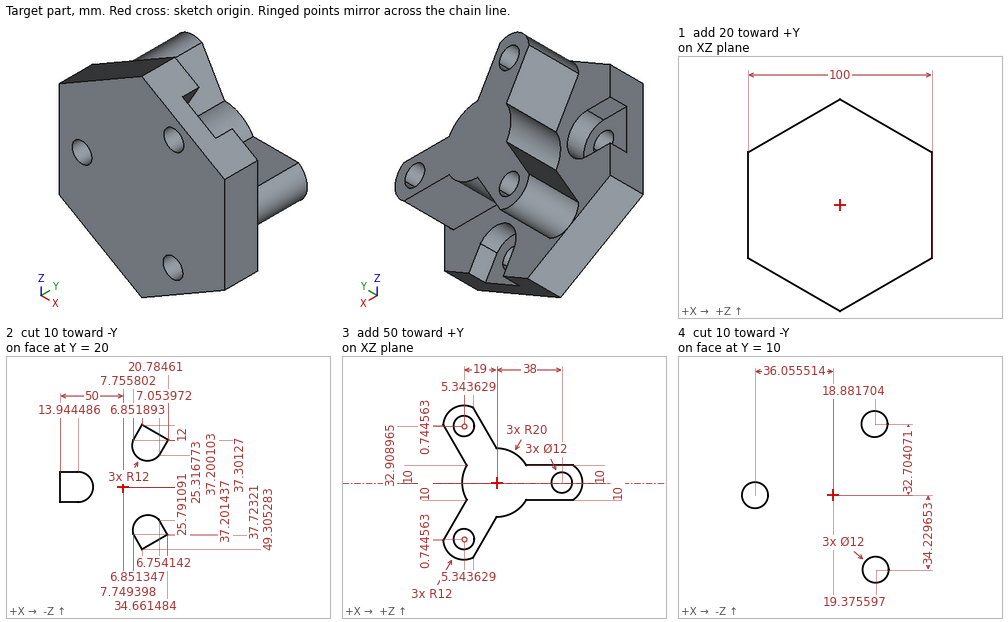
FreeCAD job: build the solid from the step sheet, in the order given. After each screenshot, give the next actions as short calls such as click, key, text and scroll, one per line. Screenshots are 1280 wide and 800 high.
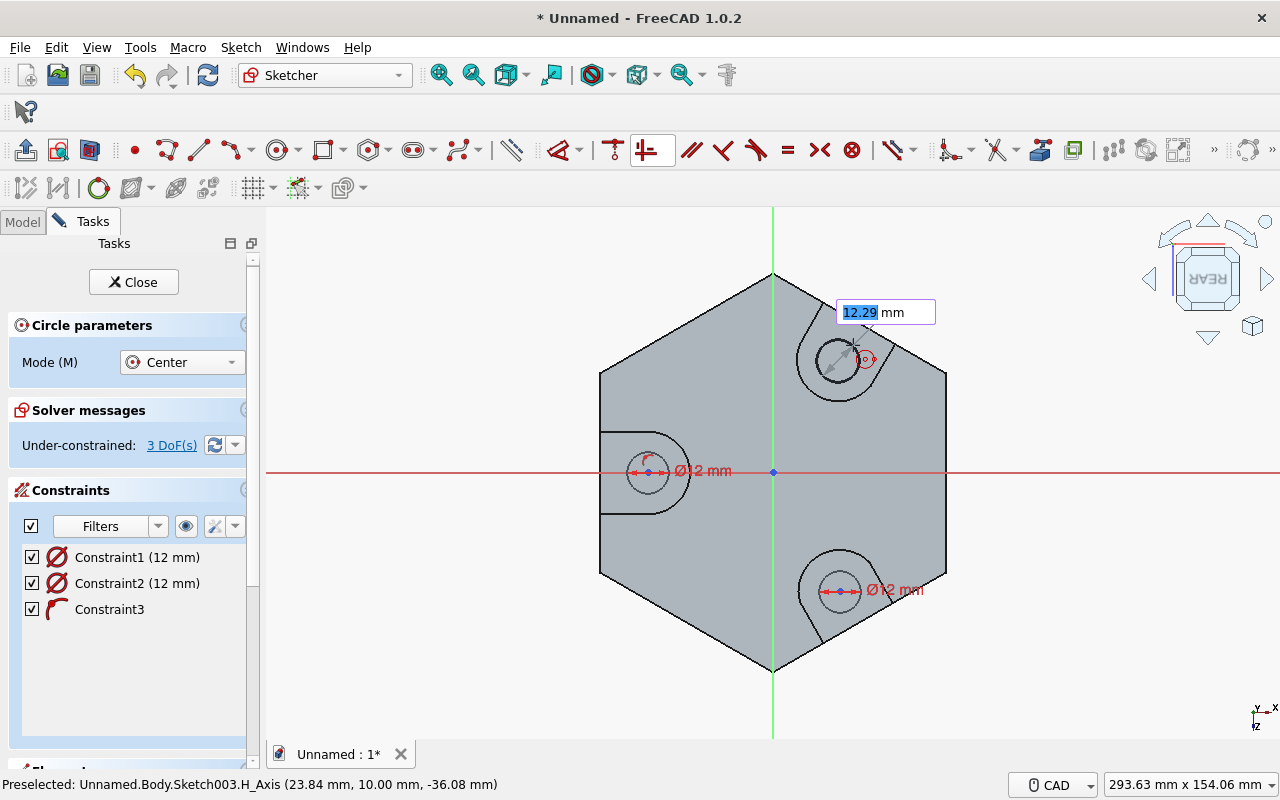
text(12)
key(Return)
key(Escape)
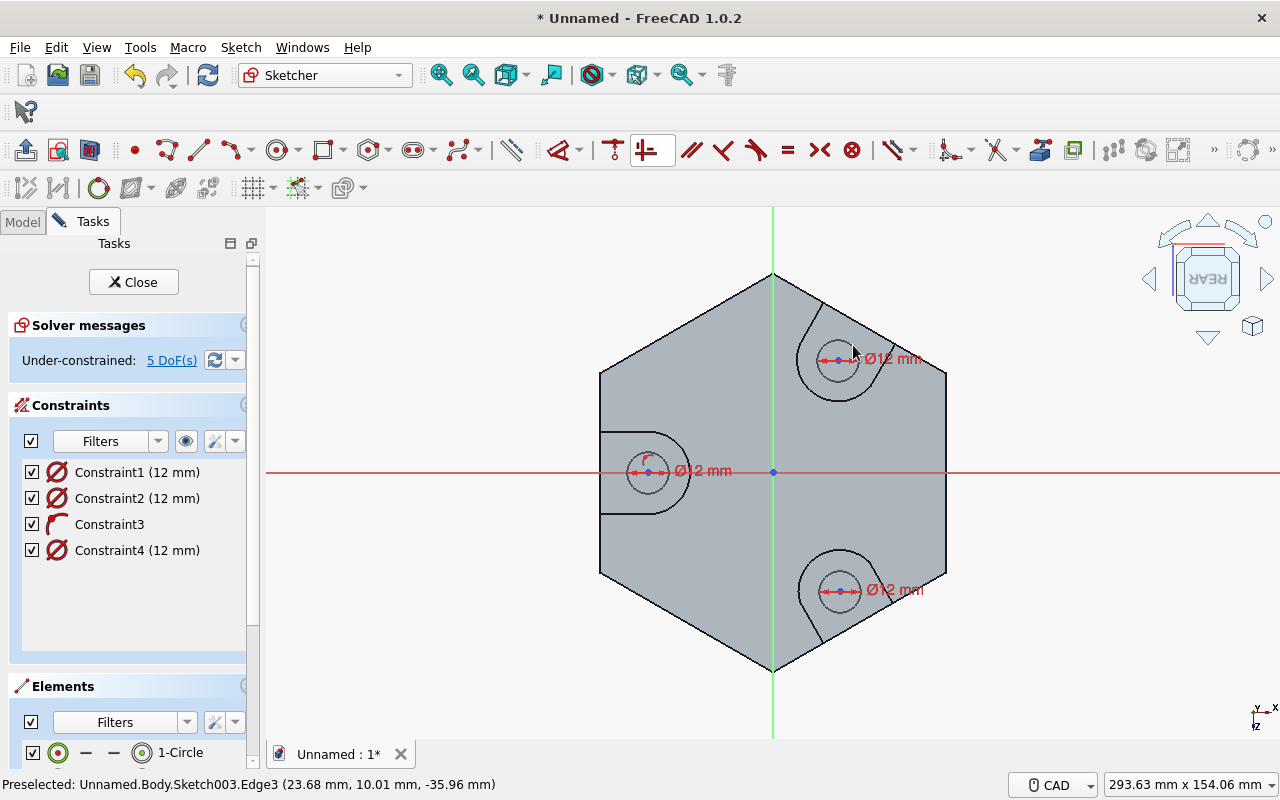
click(558, 150)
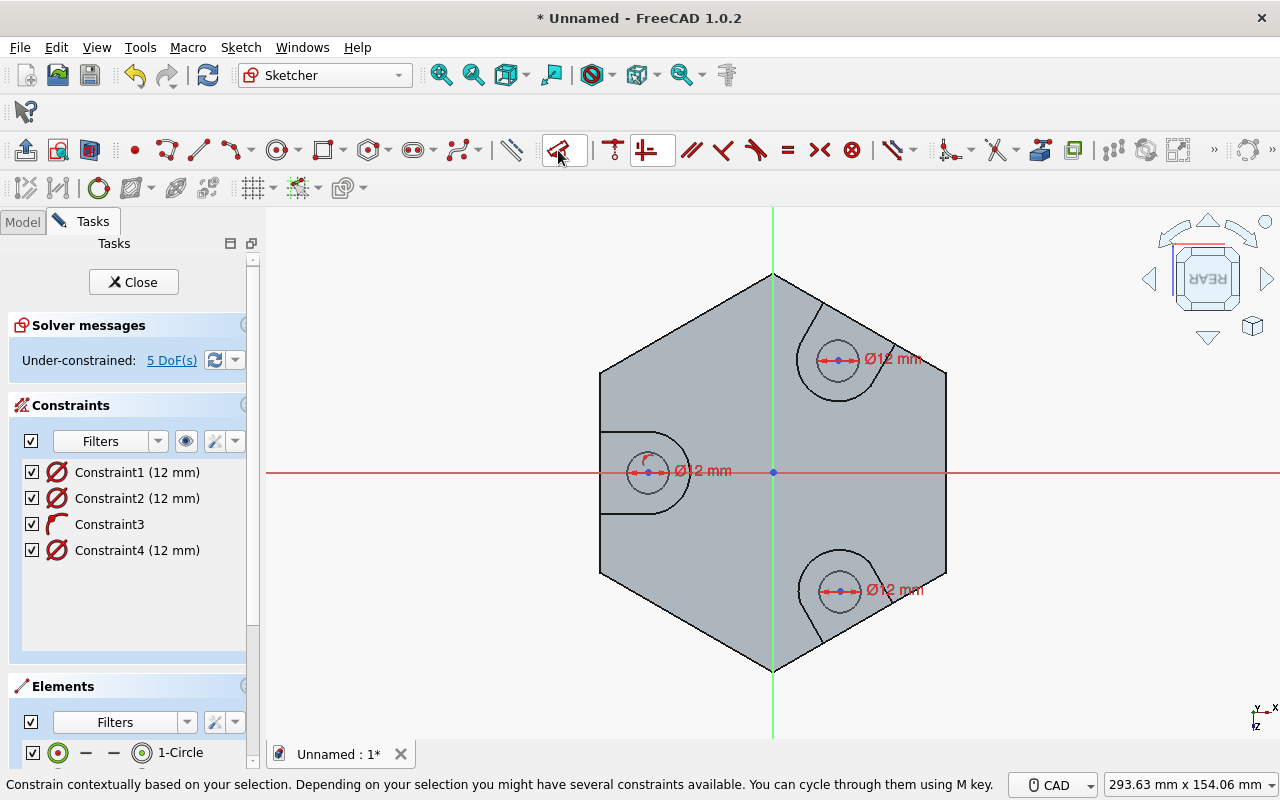
click(840, 592)
click(806, 626)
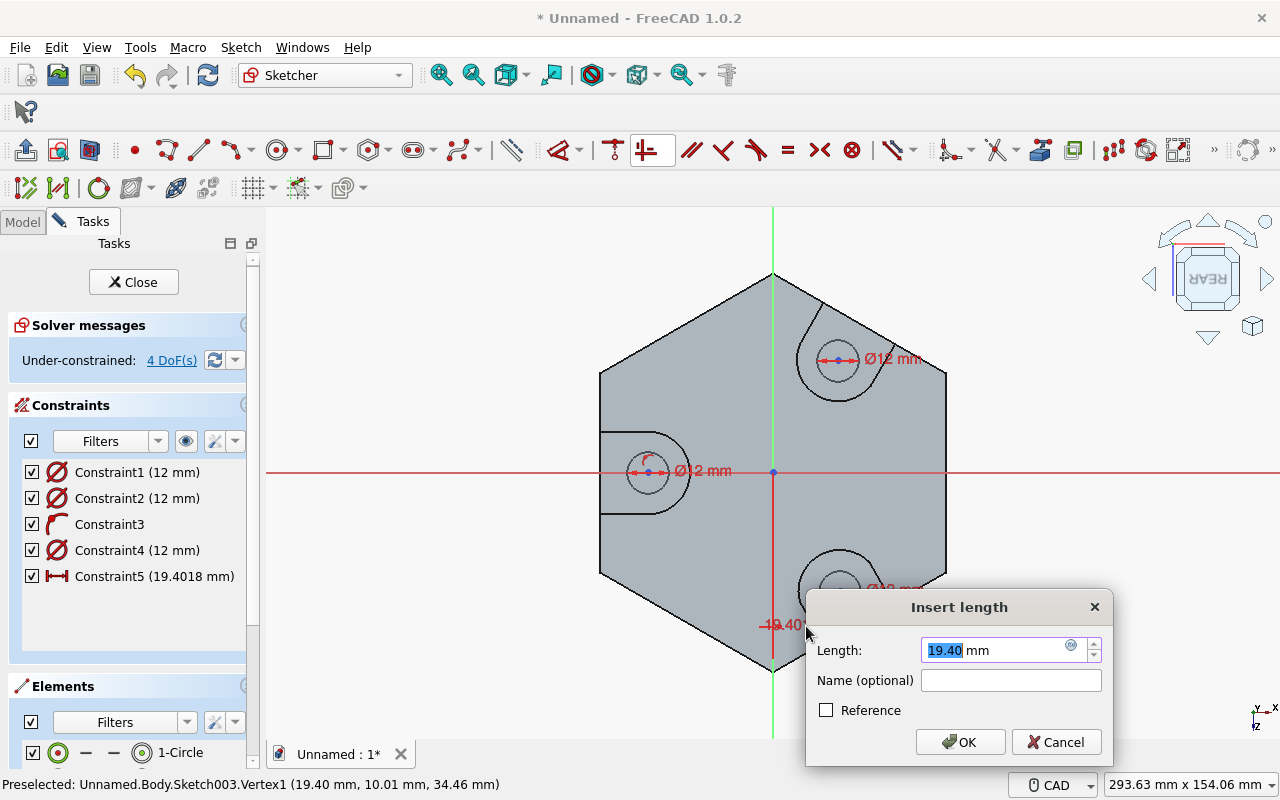
text(19.375597)
key(Return)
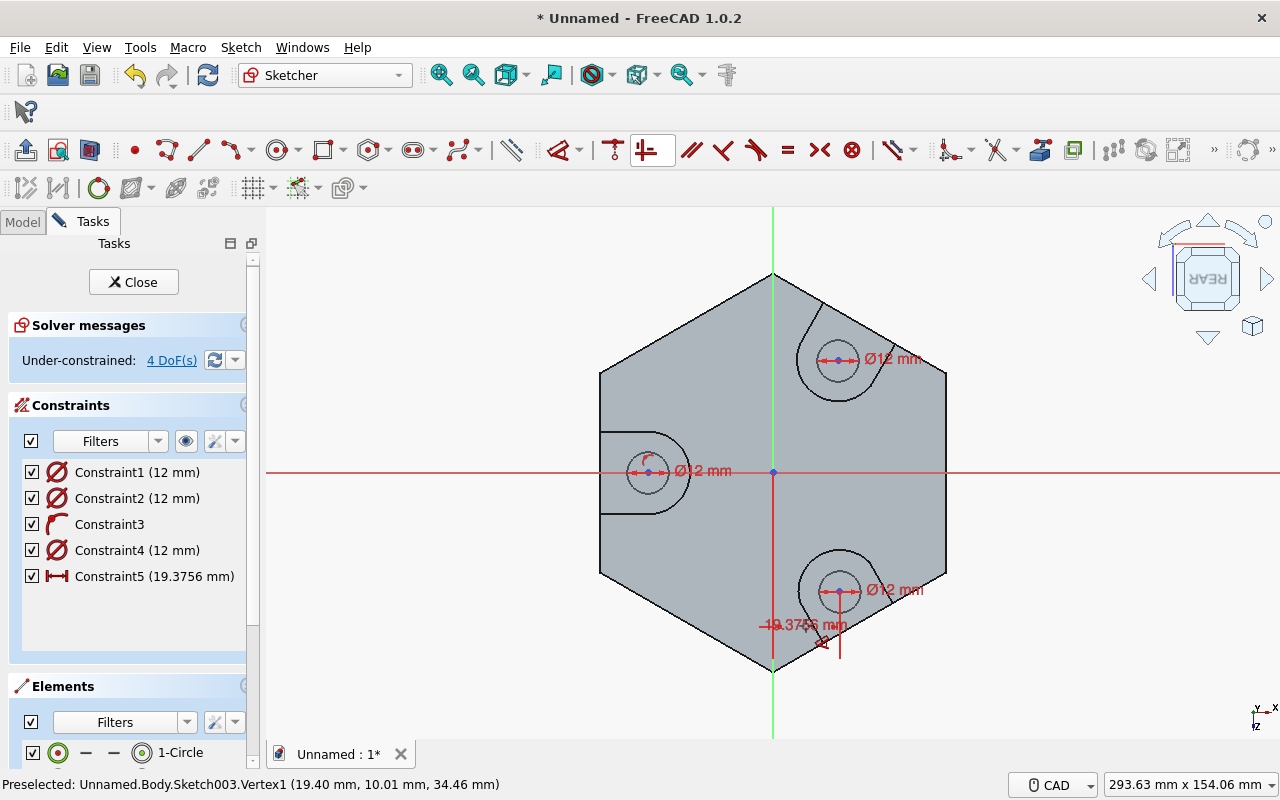
click(840, 592)
click(874, 532)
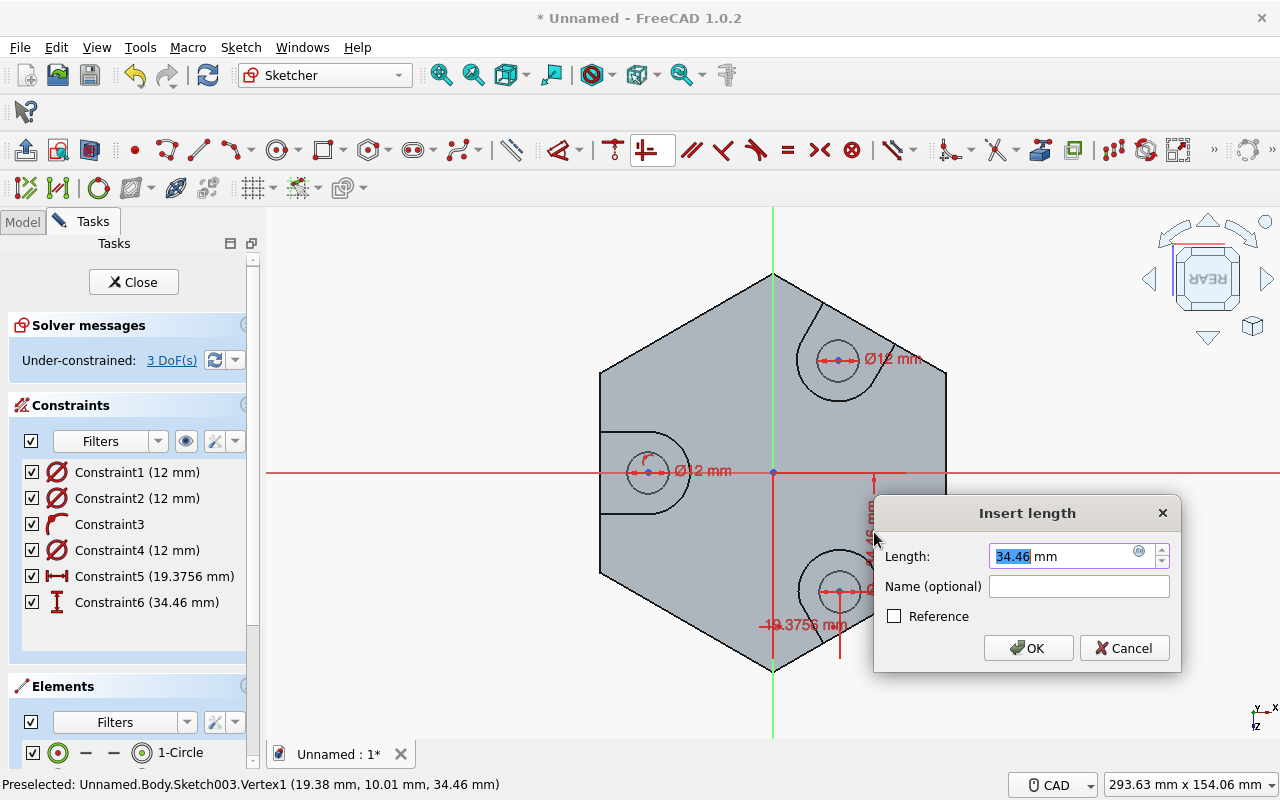
text(34.229653)
key(Return)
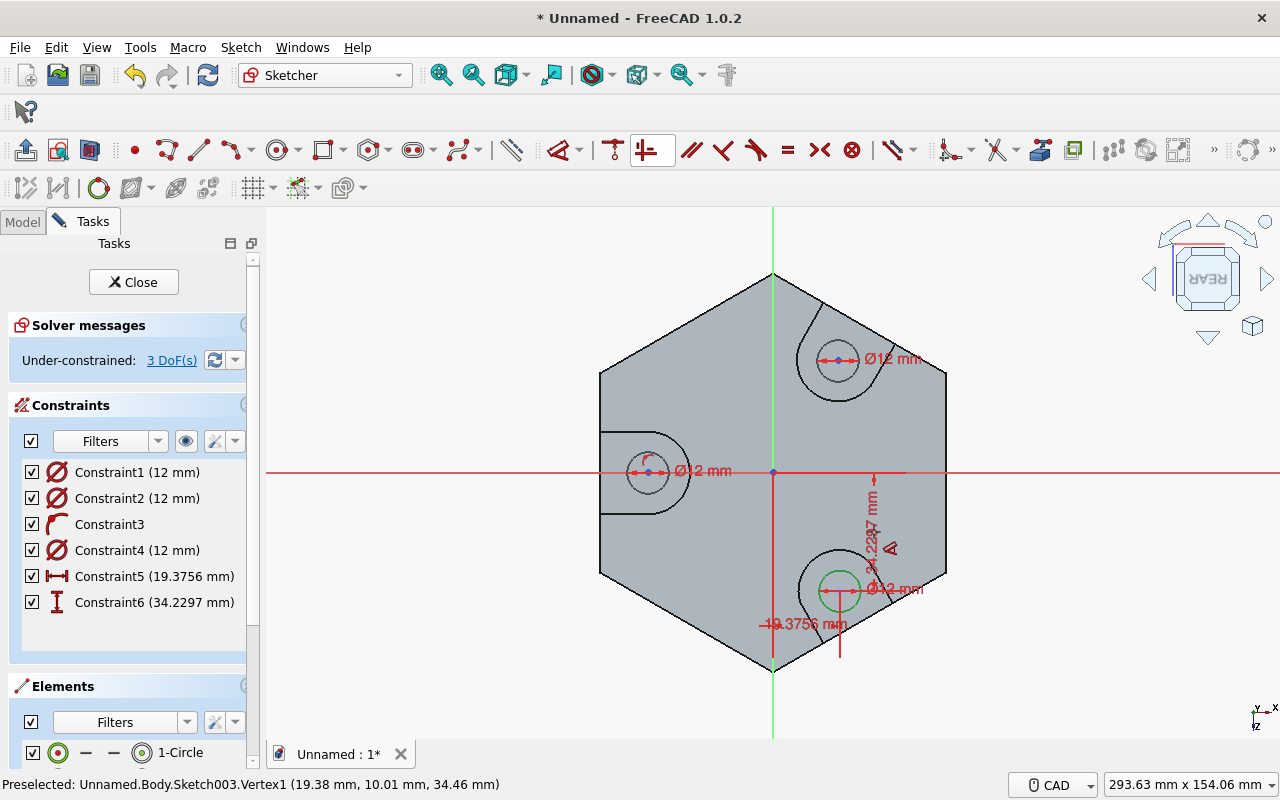
click(648, 473)
click(711, 439)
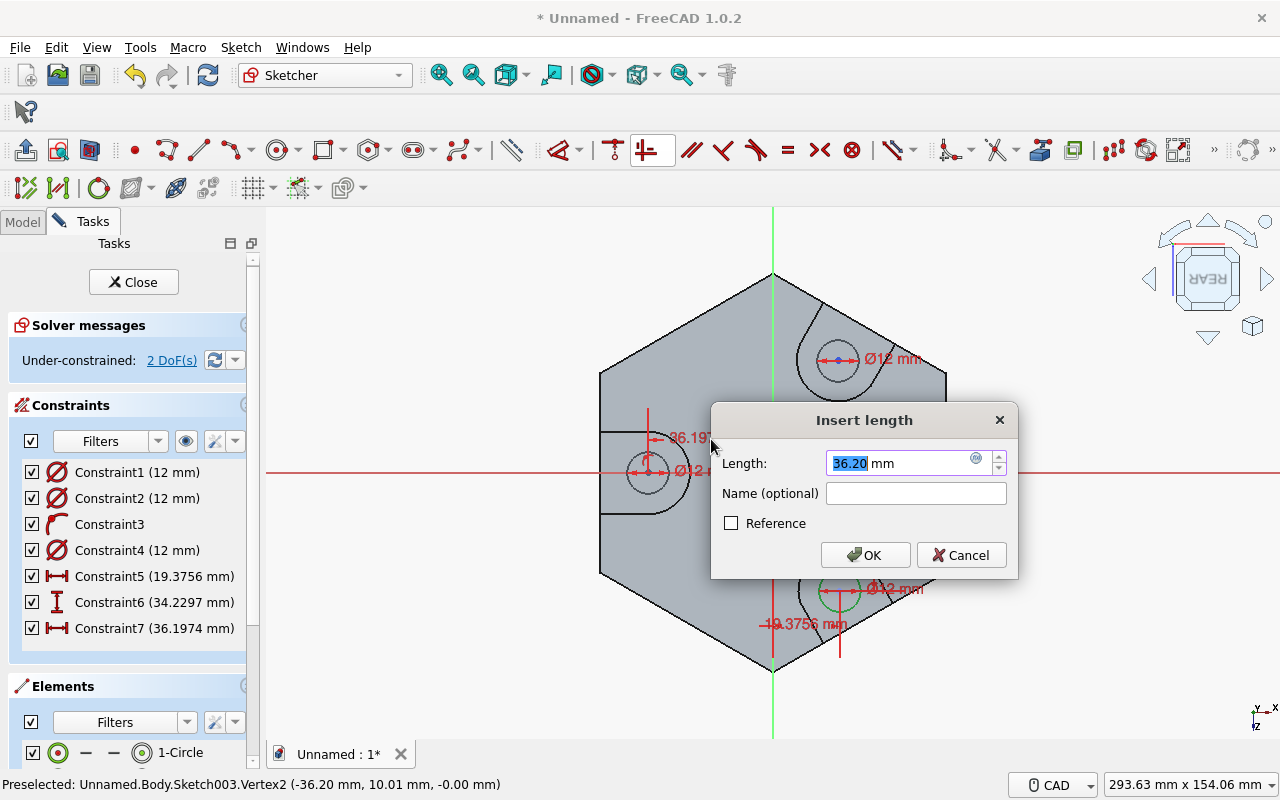
text(36.055514)
key(Return)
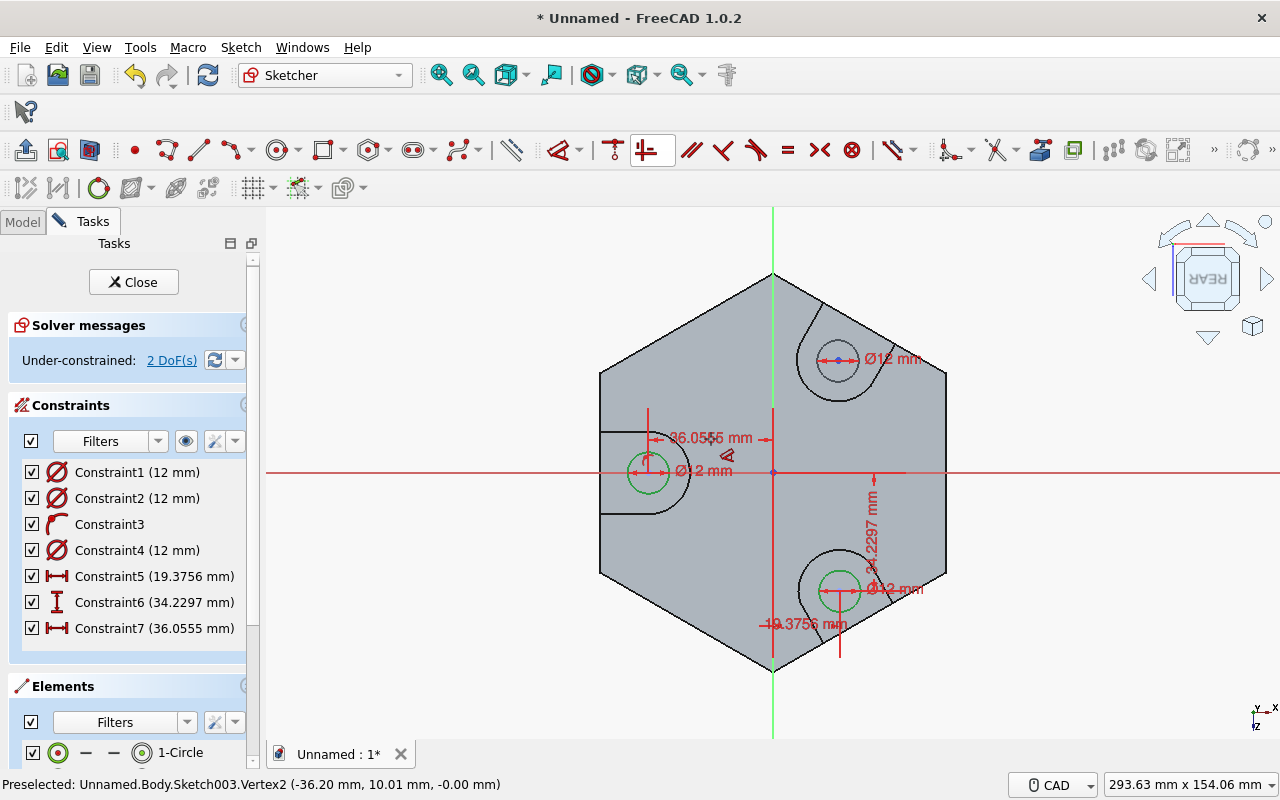
click(838, 361)
click(806, 327)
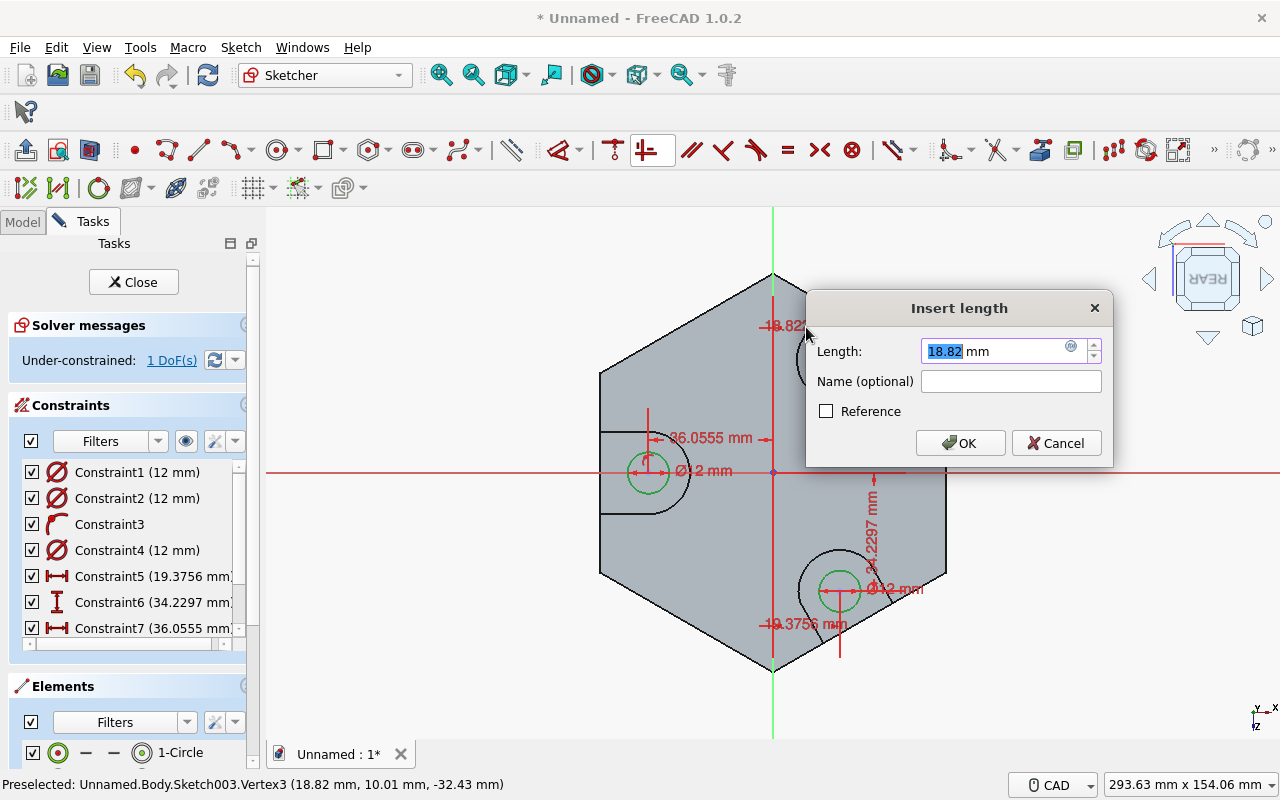
text(18.881704)
key(Return)